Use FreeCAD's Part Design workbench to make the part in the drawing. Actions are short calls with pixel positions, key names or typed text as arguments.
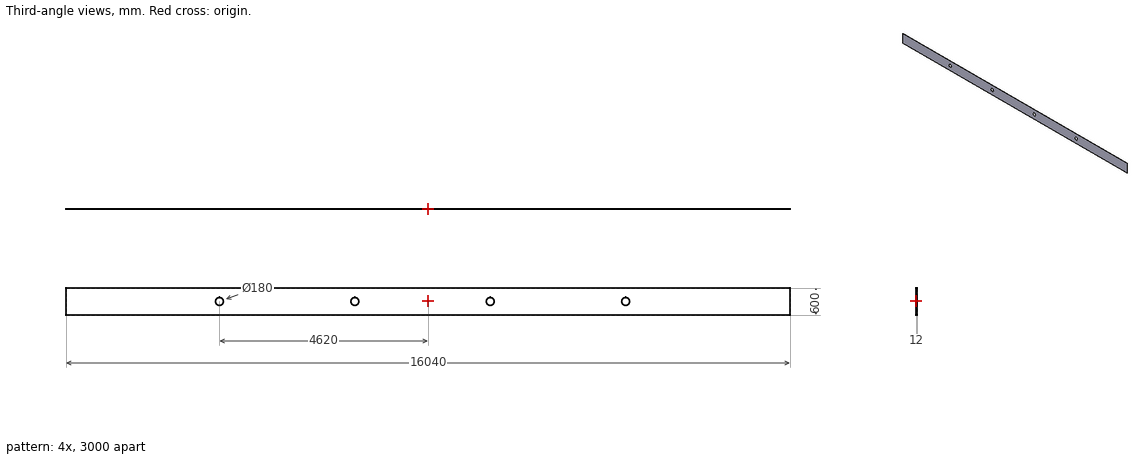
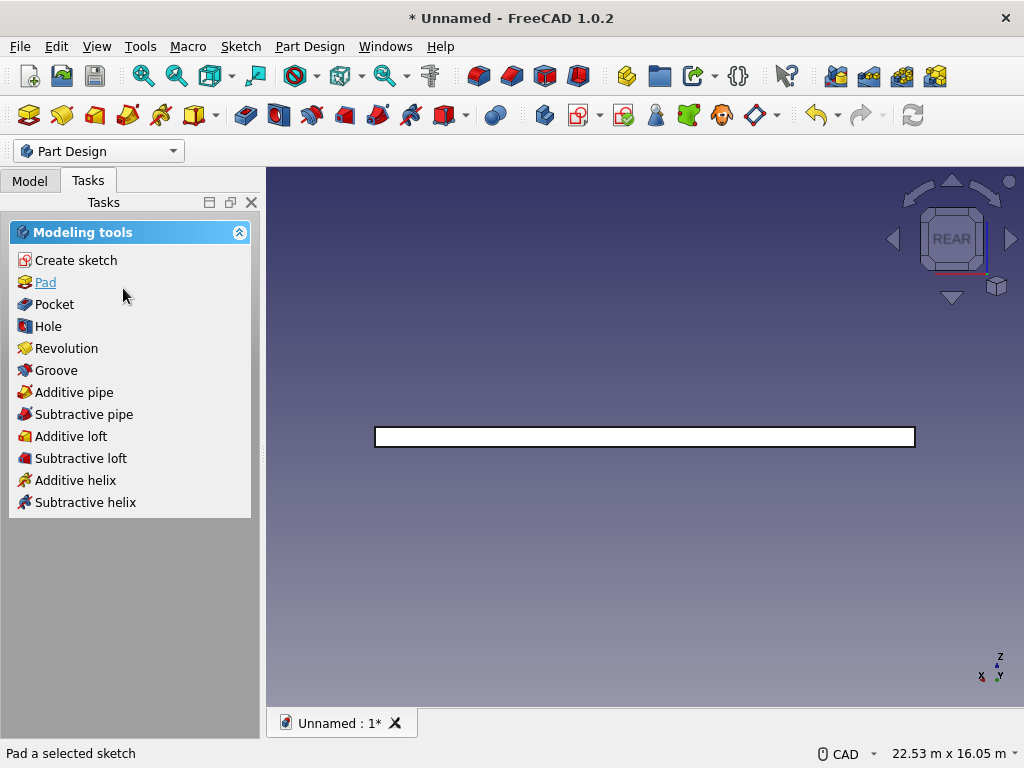
click(246, 116)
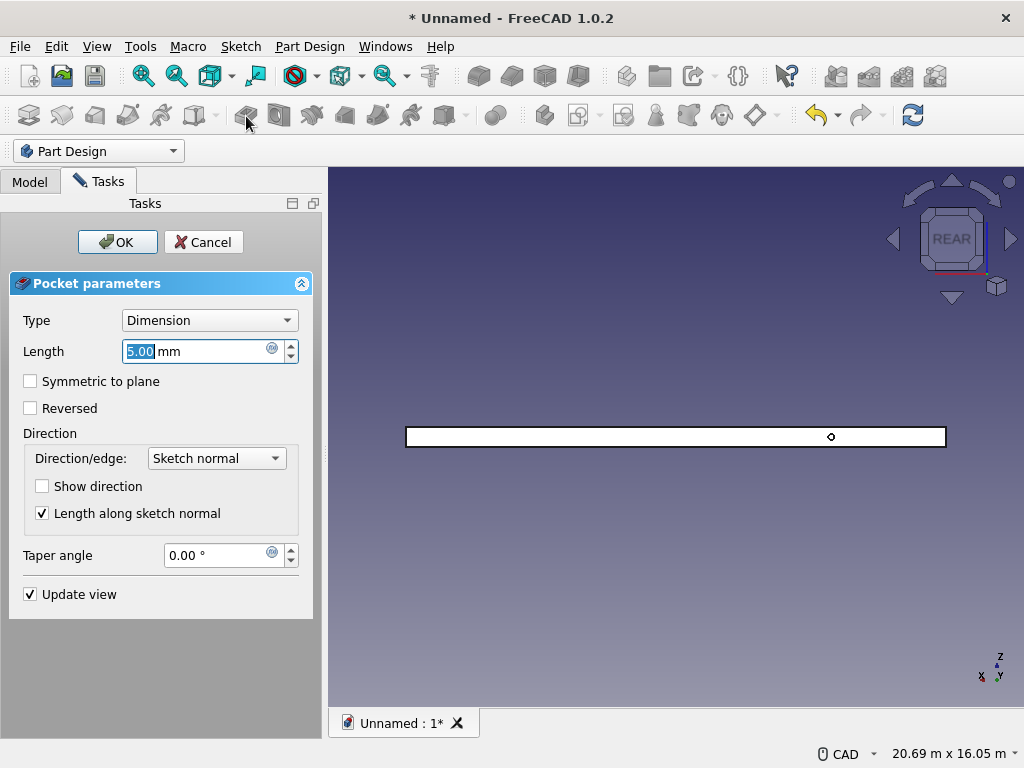
click(210, 320)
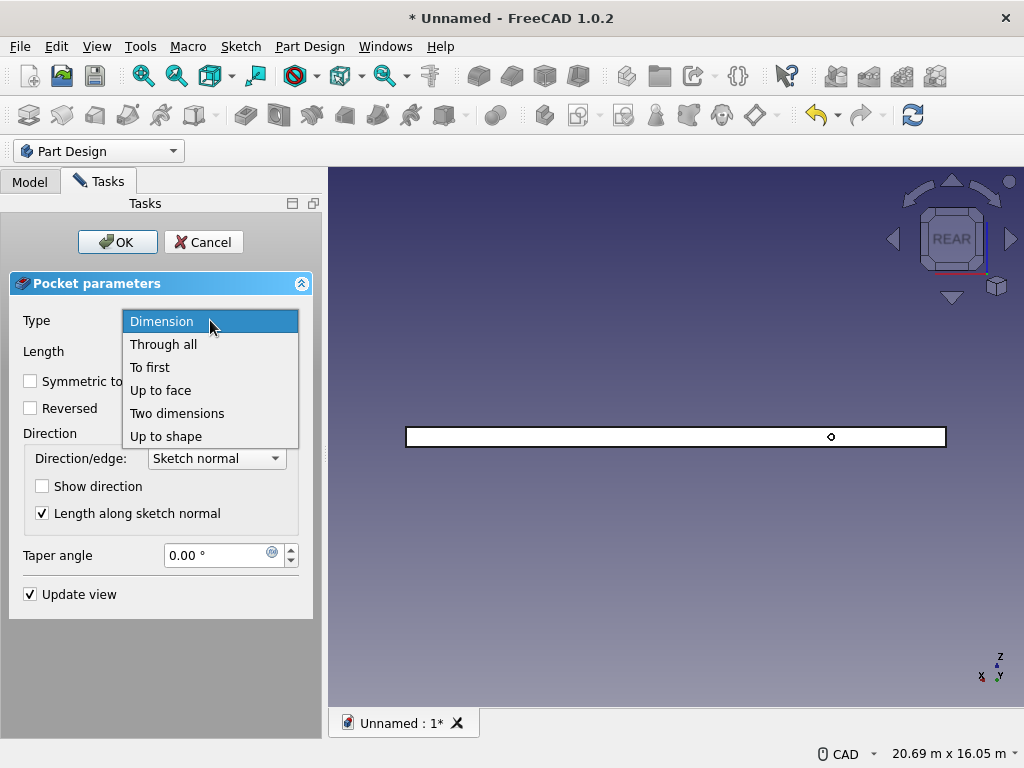
click(208, 344)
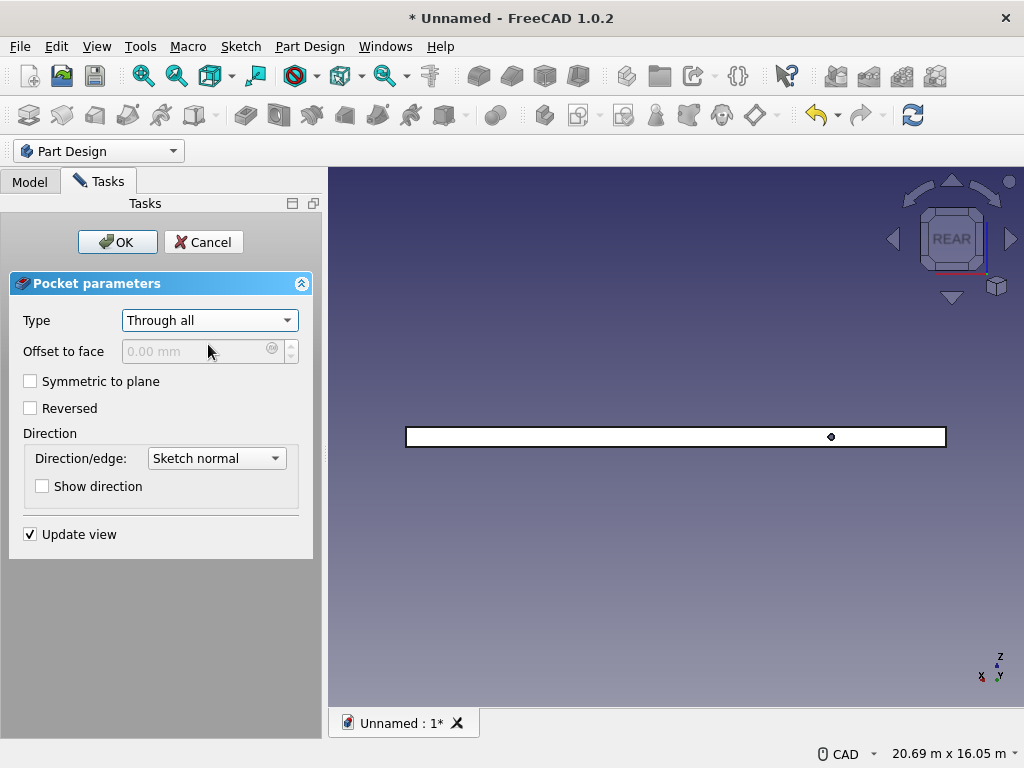
click(118, 242)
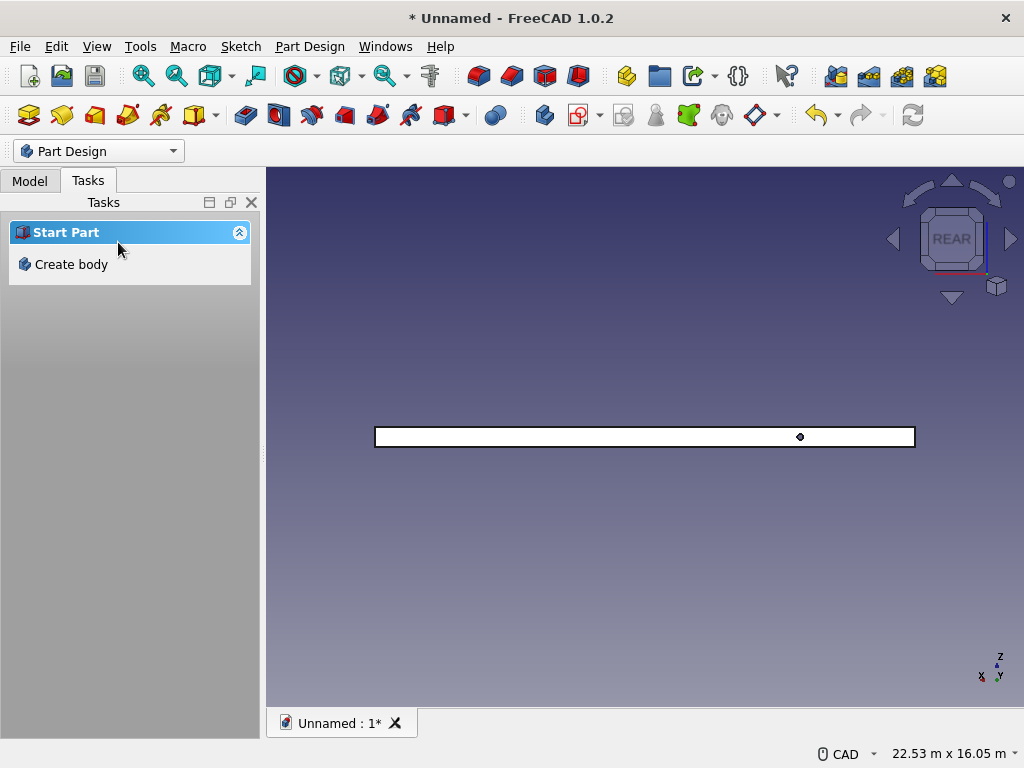
click(30, 180)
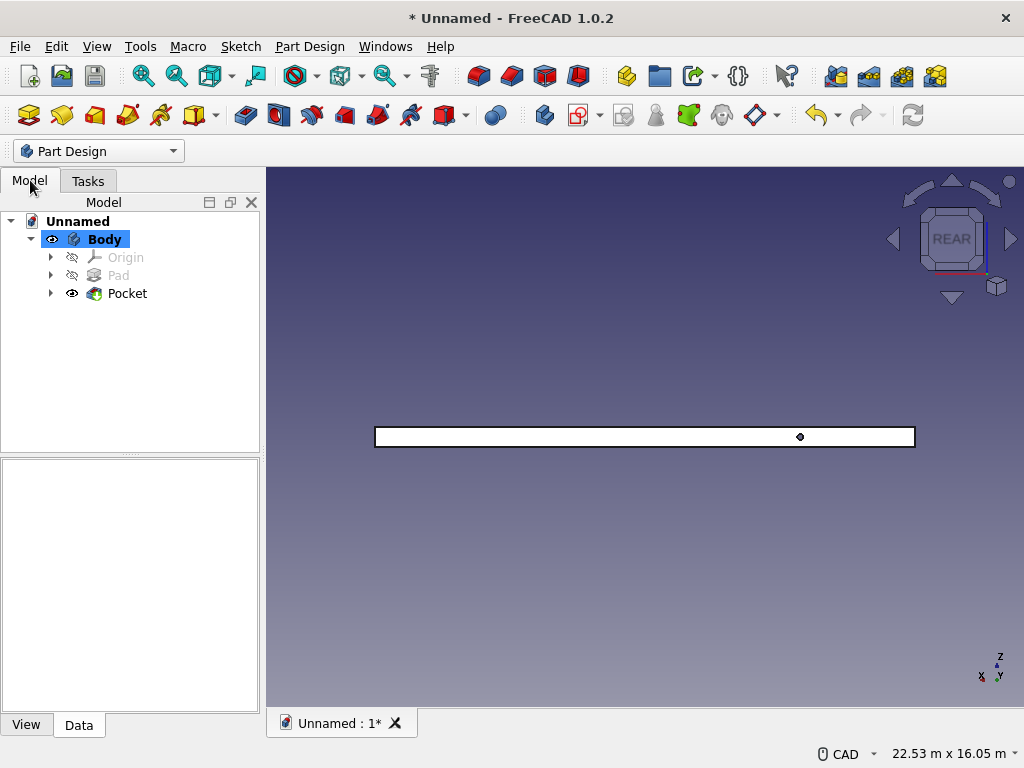
click(117, 293)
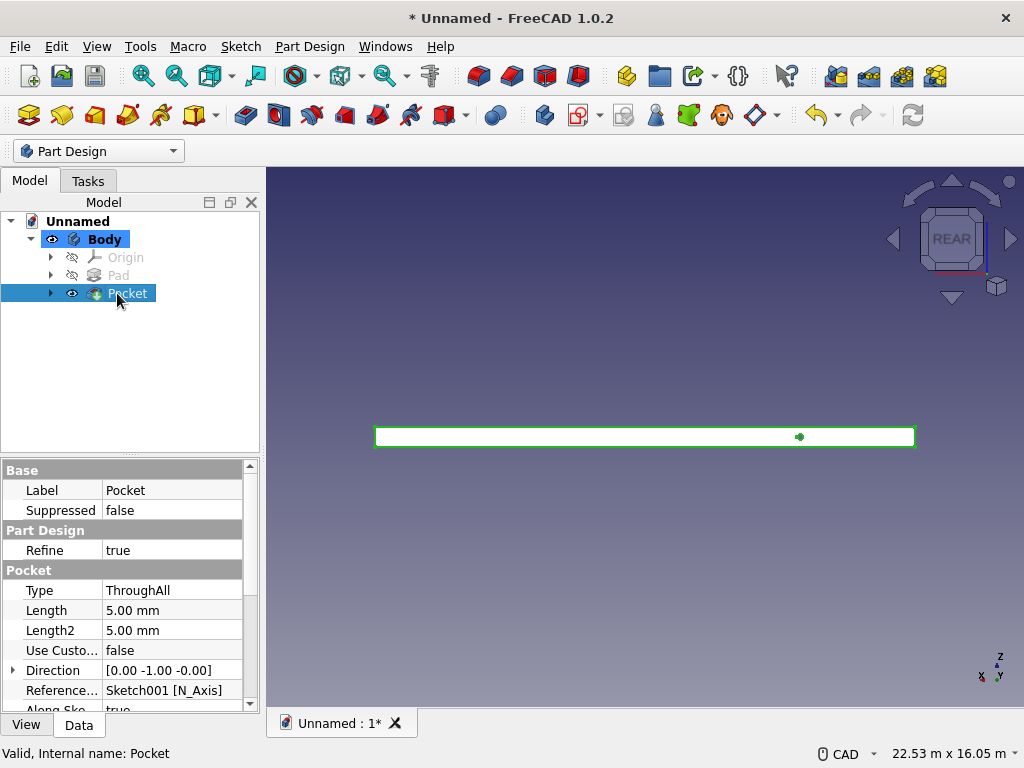
click(869, 76)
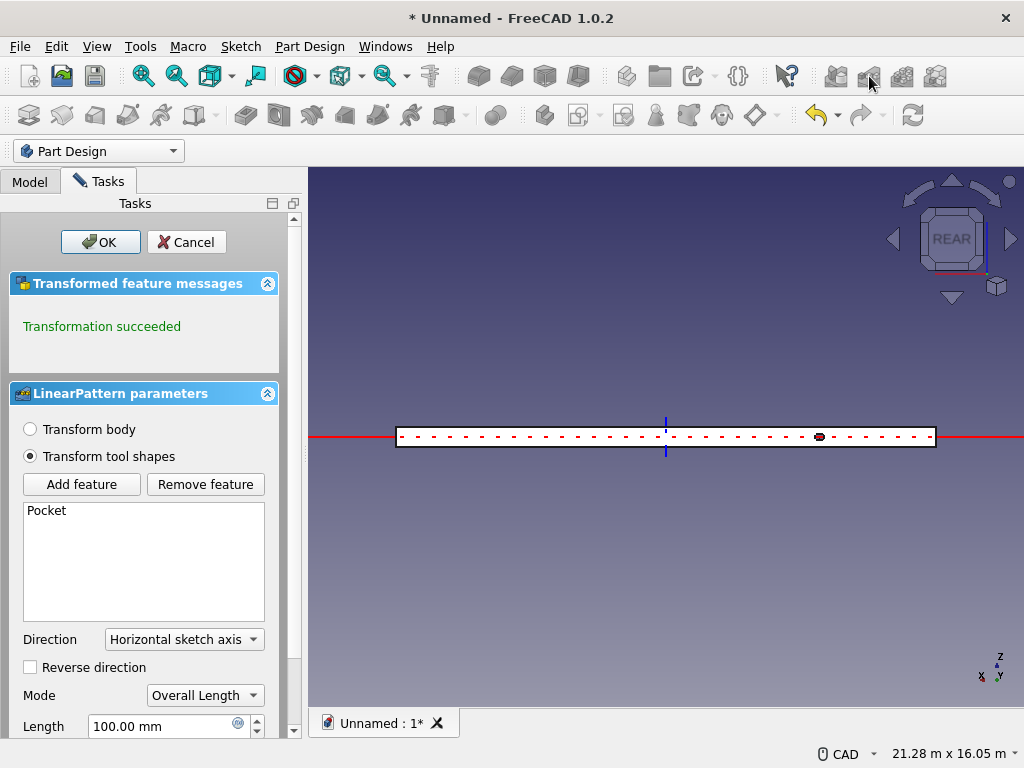
click(185, 640)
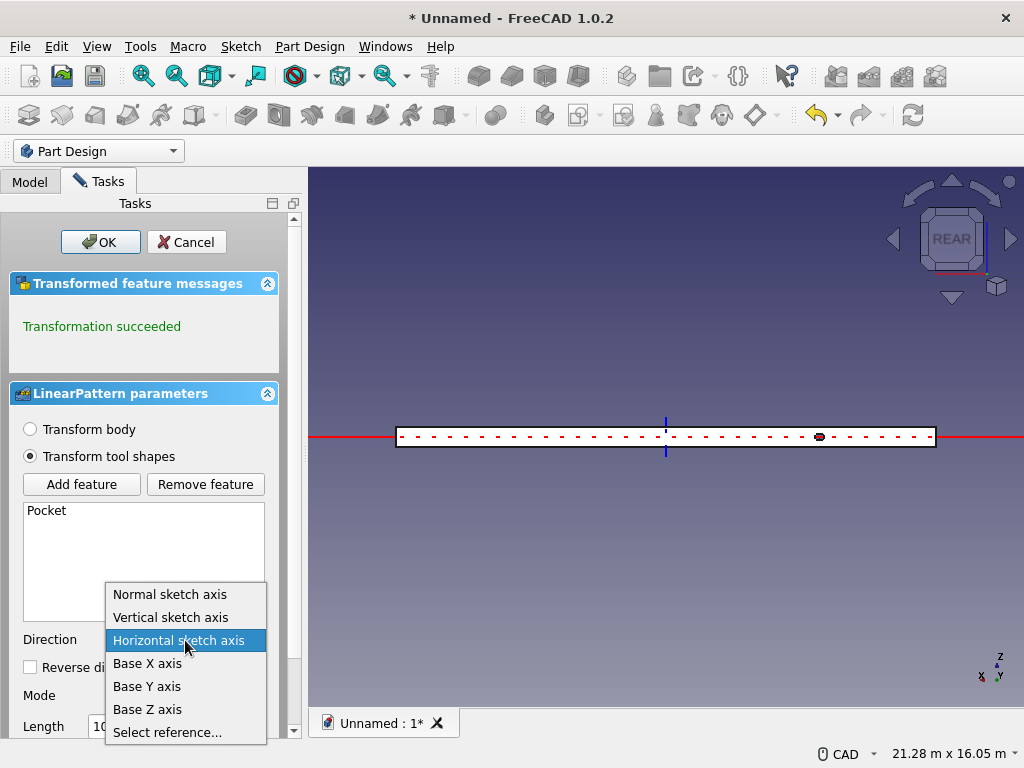
click(184, 664)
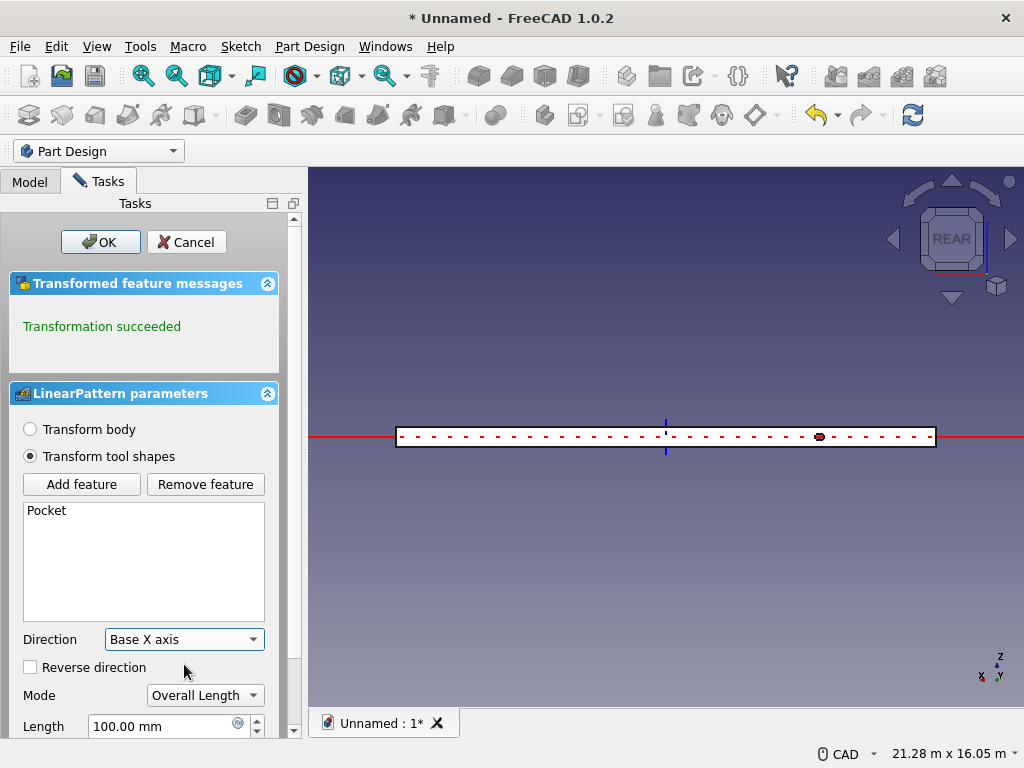
click(206, 696)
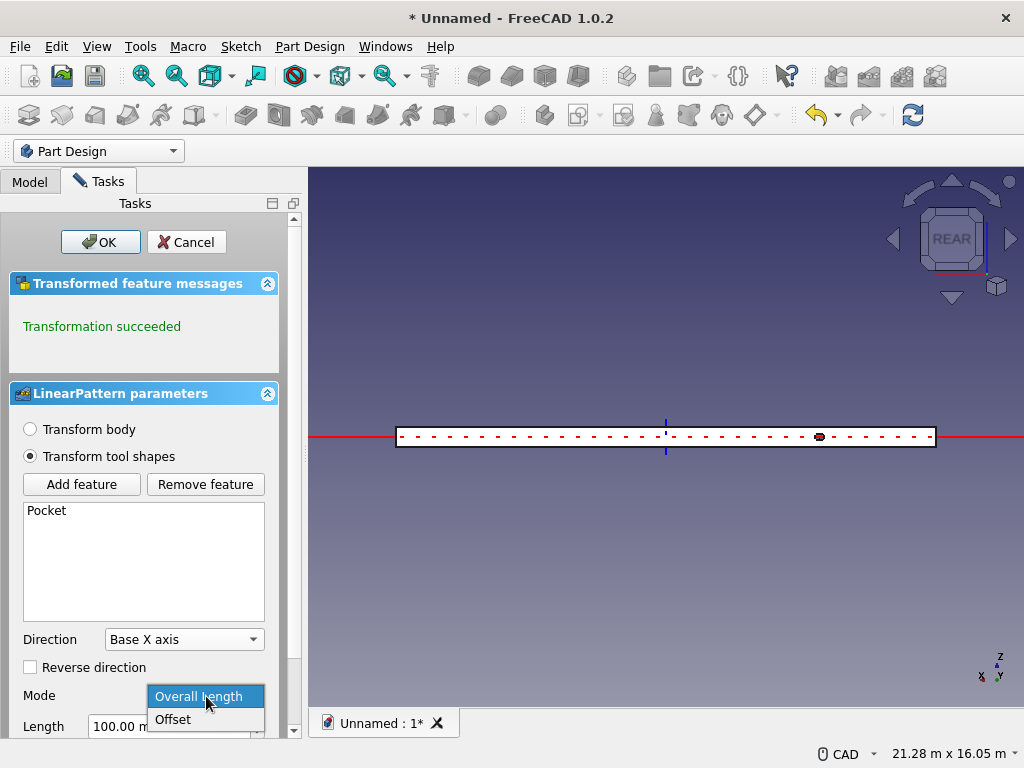
click(204, 720)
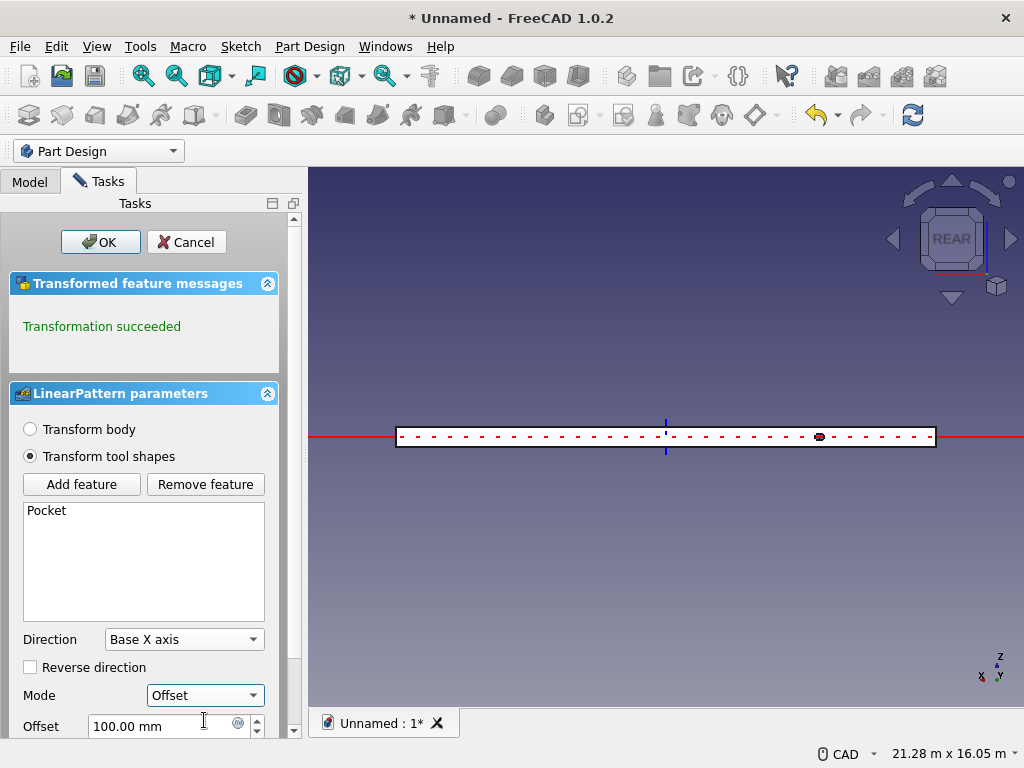
scroll(294, 476, down, 2)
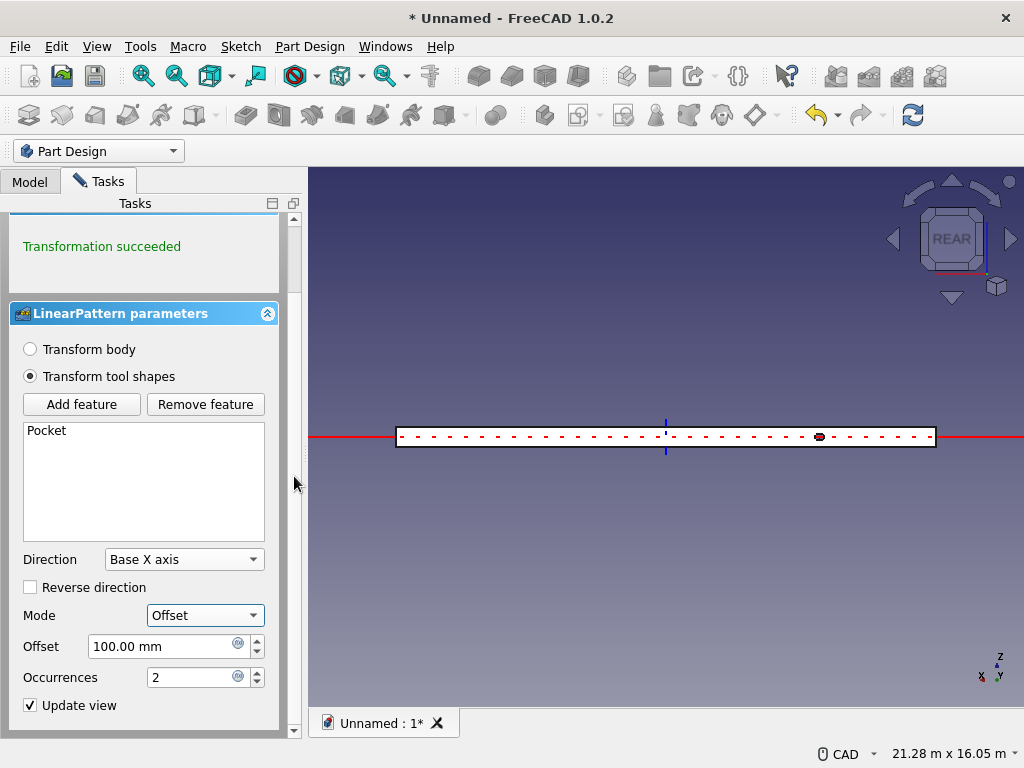
triple_click(170, 646)